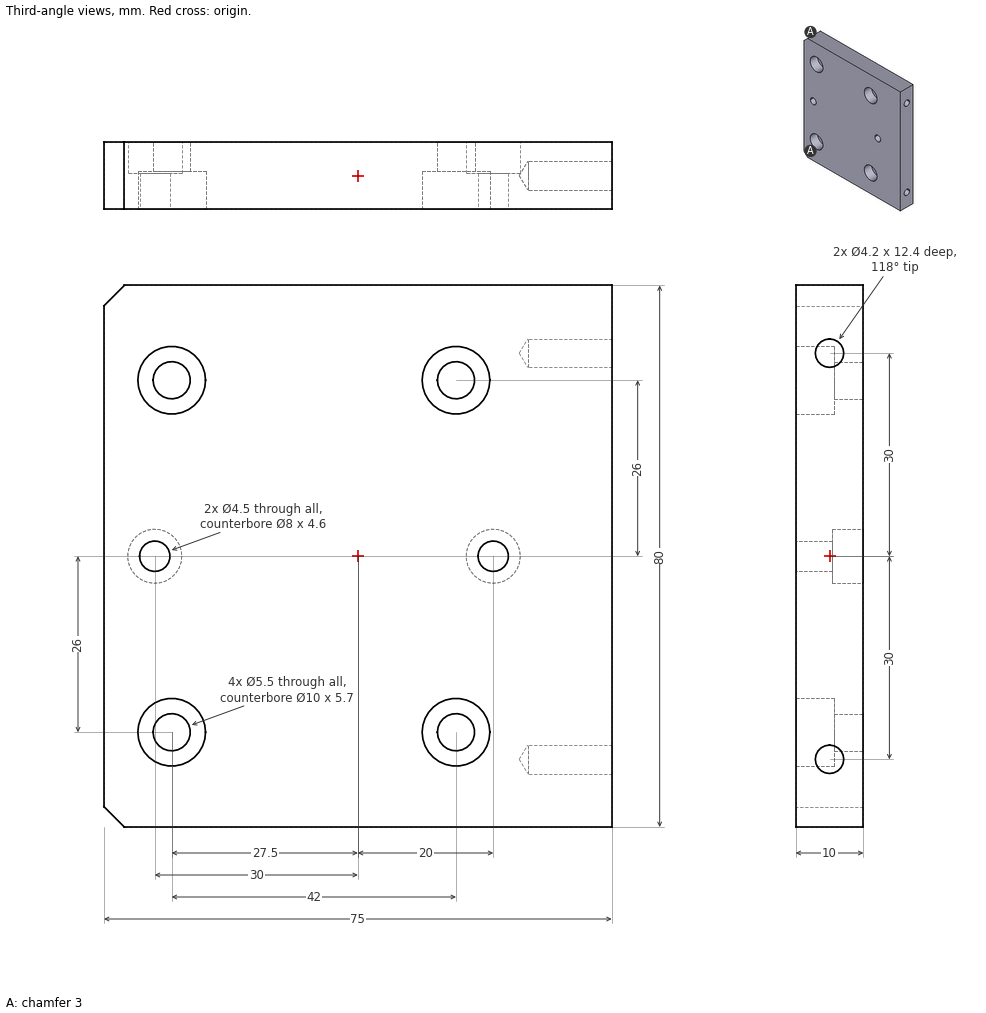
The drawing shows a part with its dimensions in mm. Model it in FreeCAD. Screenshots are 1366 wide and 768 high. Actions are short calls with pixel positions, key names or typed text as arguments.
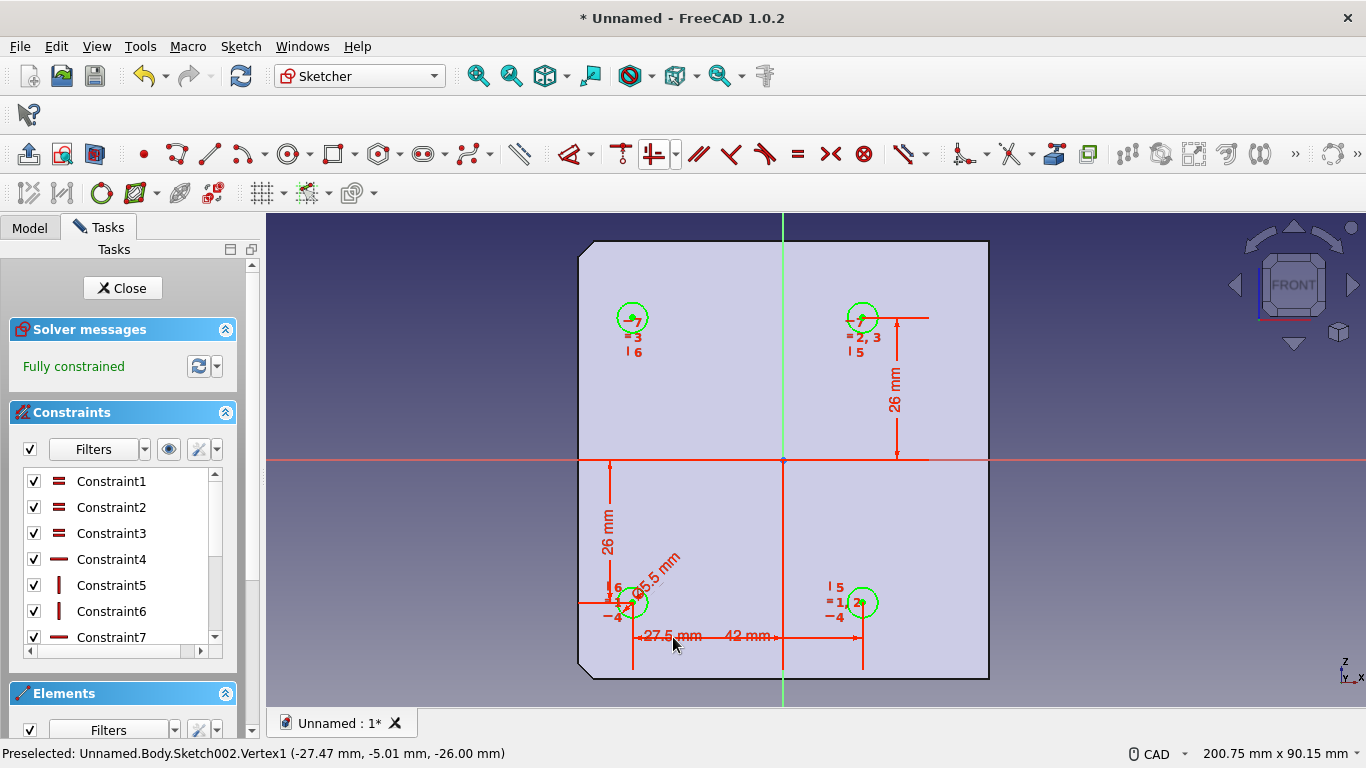
click(123, 288)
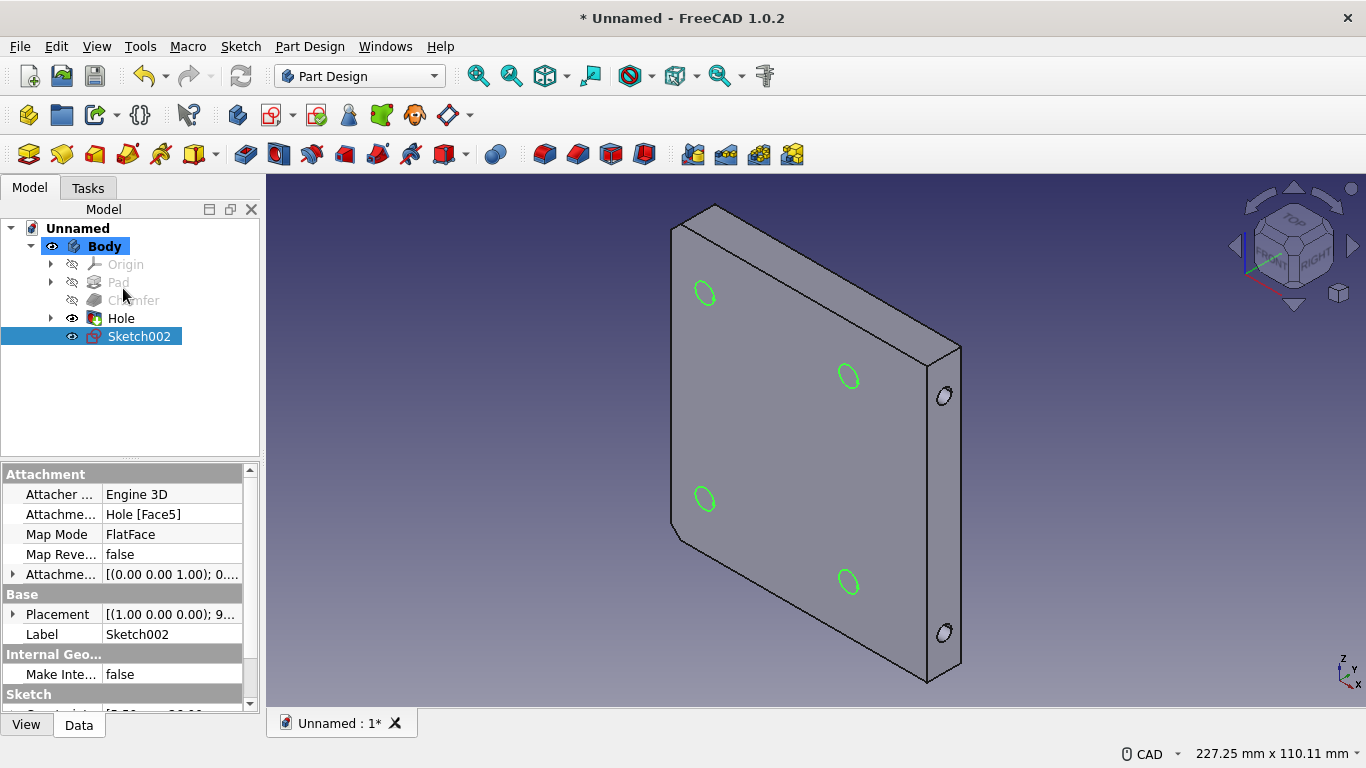
click(279, 154)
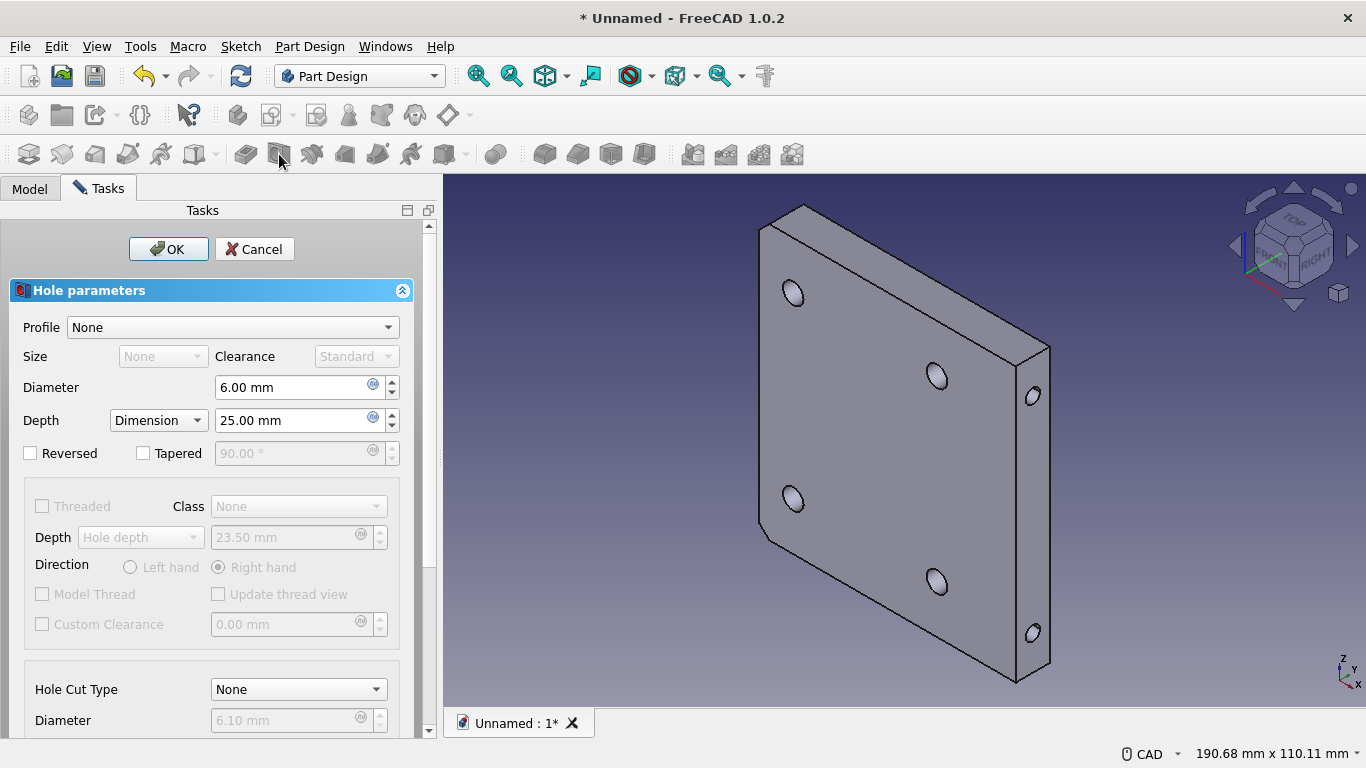
triple_click(300, 388)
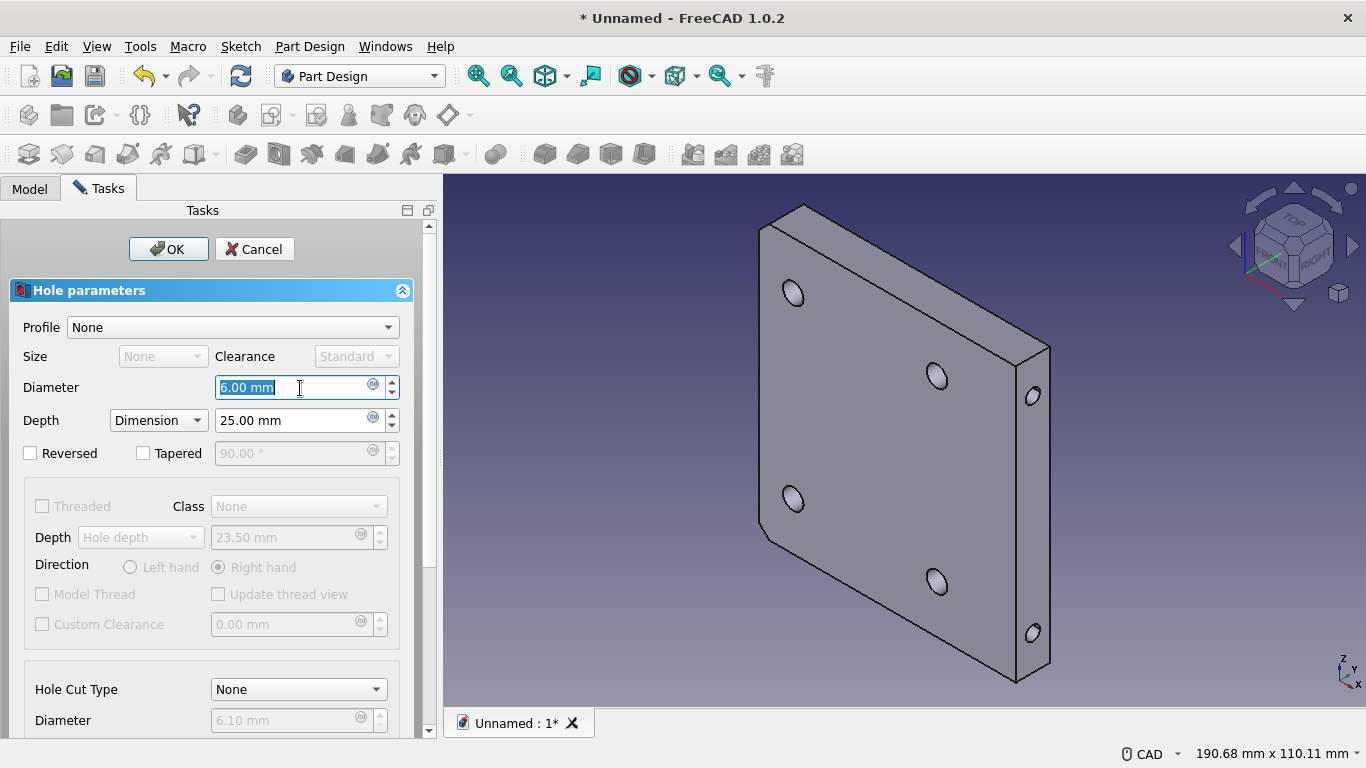
text(5.5)
key(Tab)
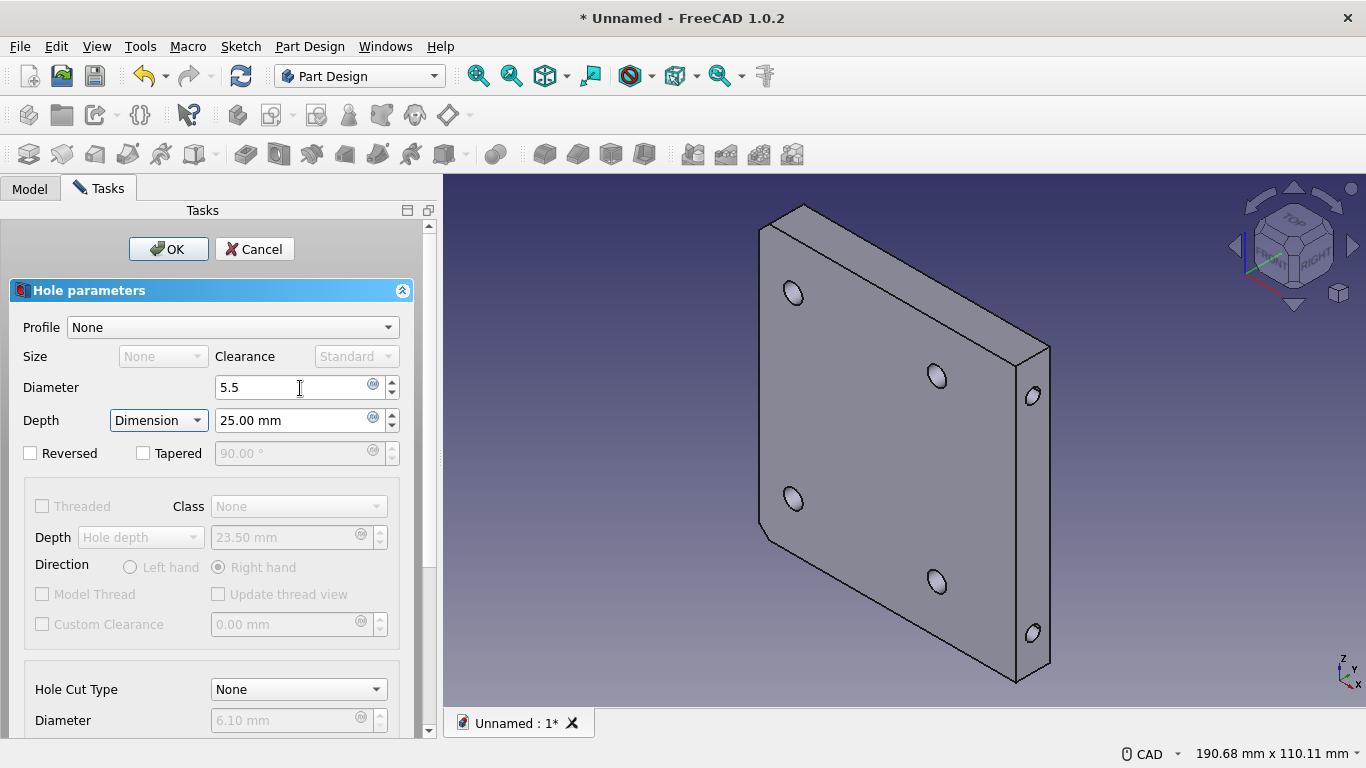
click(160, 420)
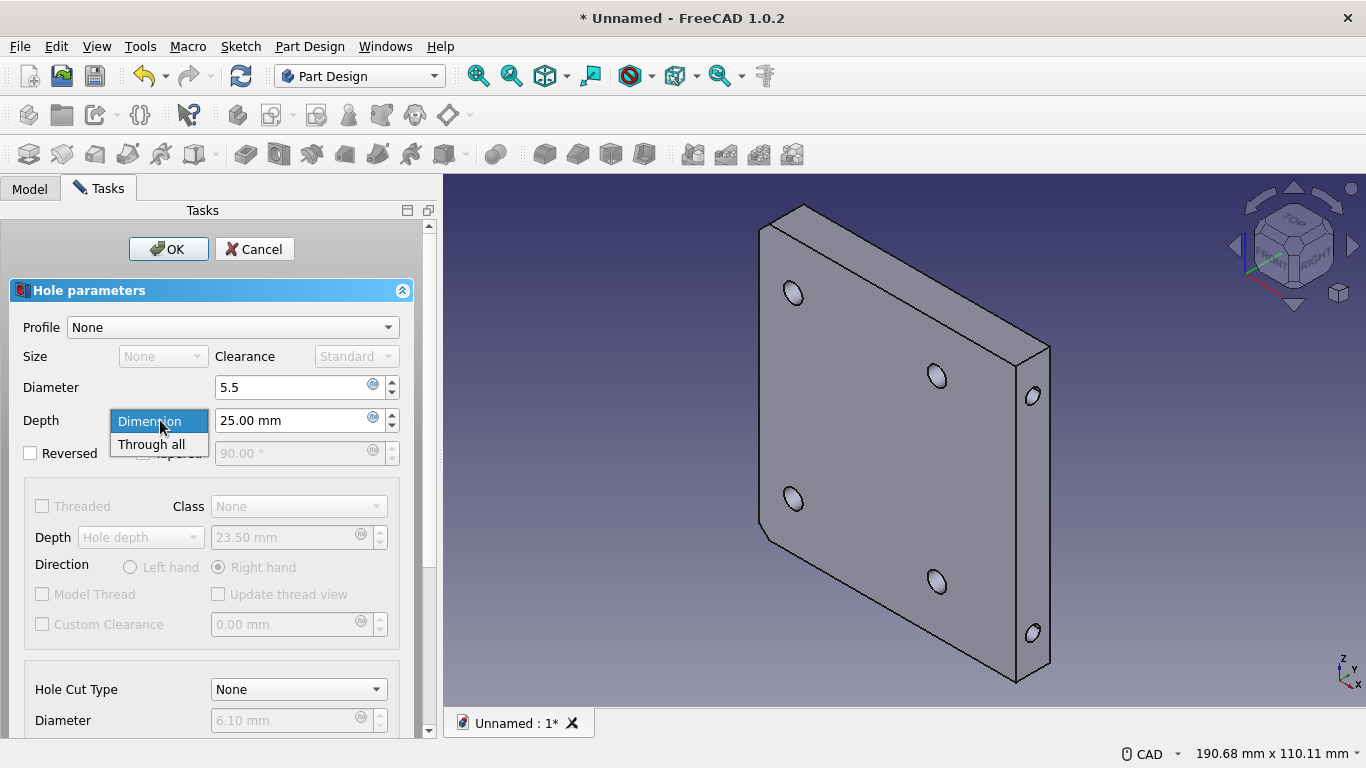
click(158, 444)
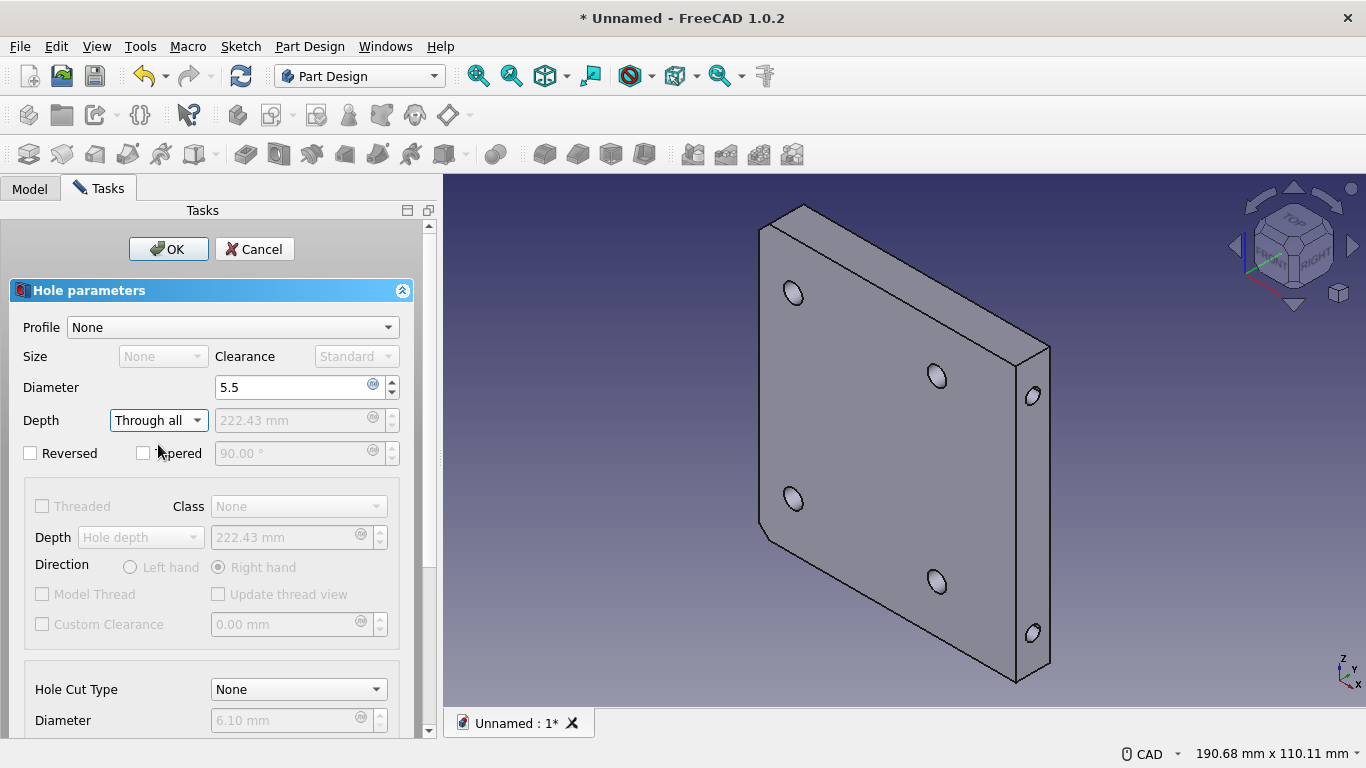
click(300, 690)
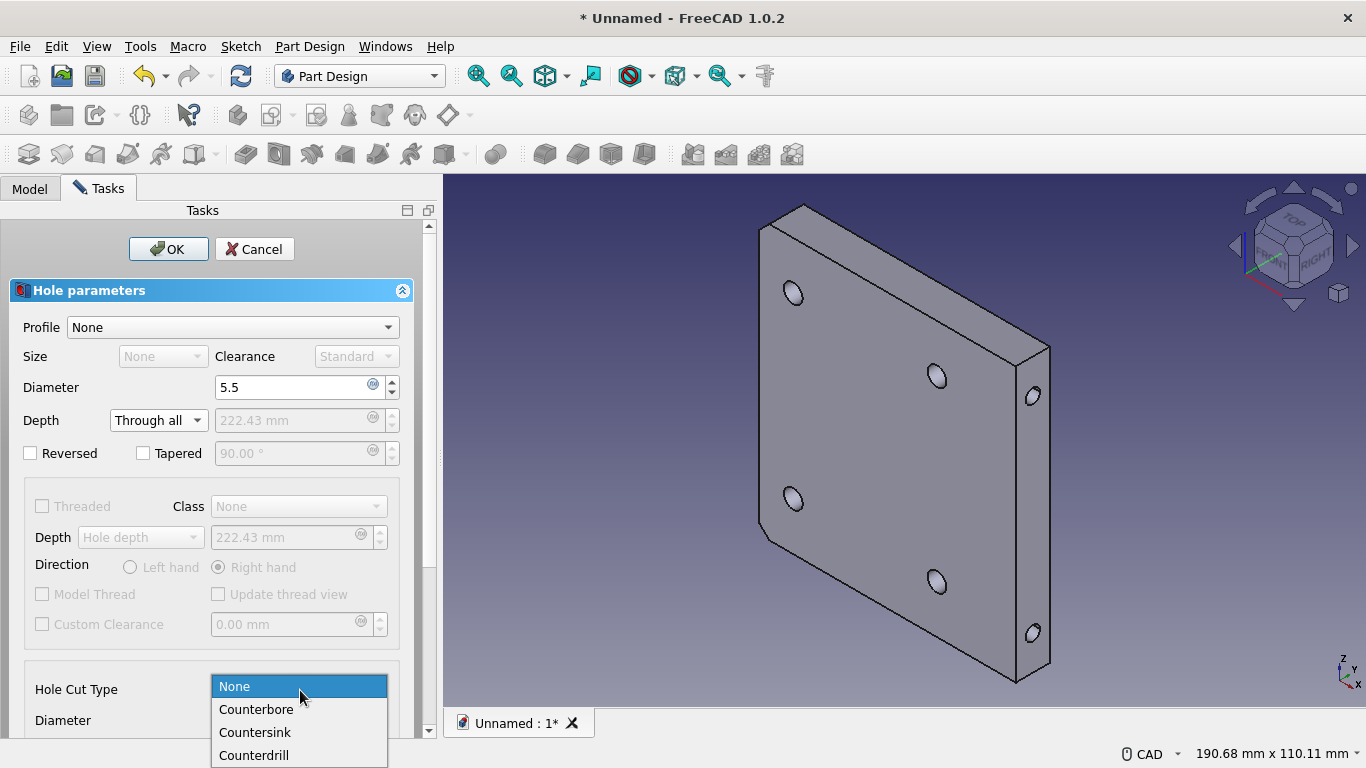
click(298, 710)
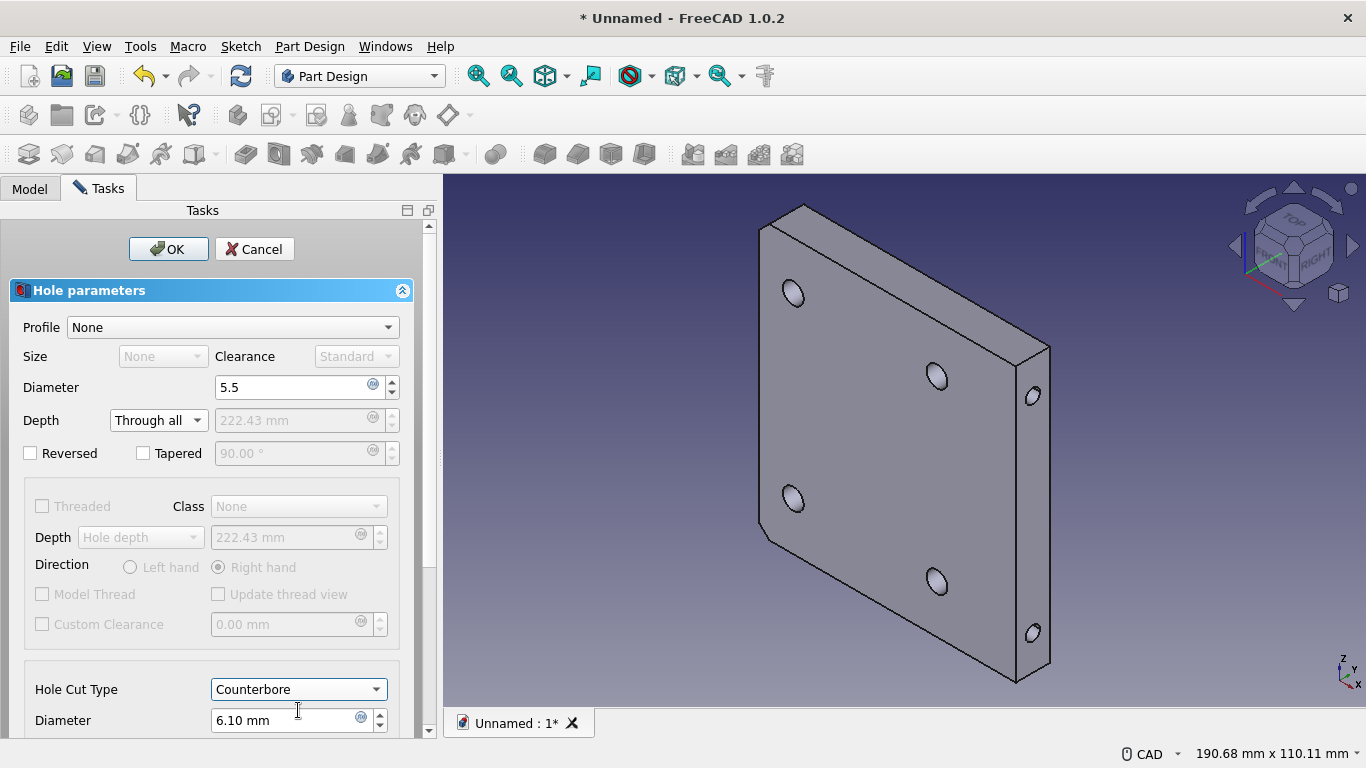
triple_click(292, 720)